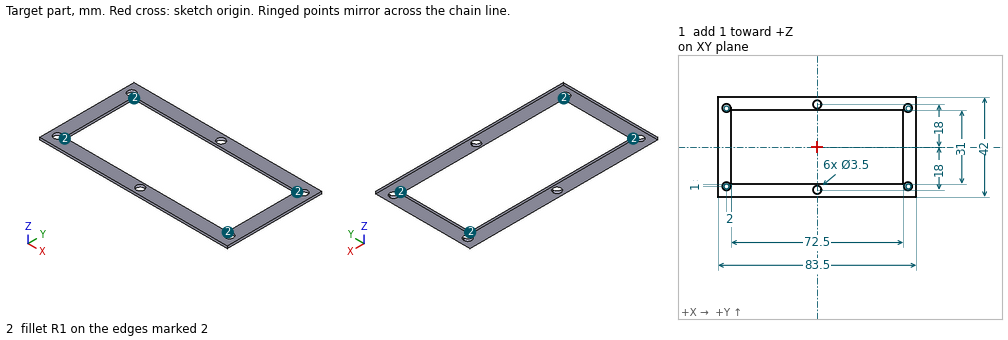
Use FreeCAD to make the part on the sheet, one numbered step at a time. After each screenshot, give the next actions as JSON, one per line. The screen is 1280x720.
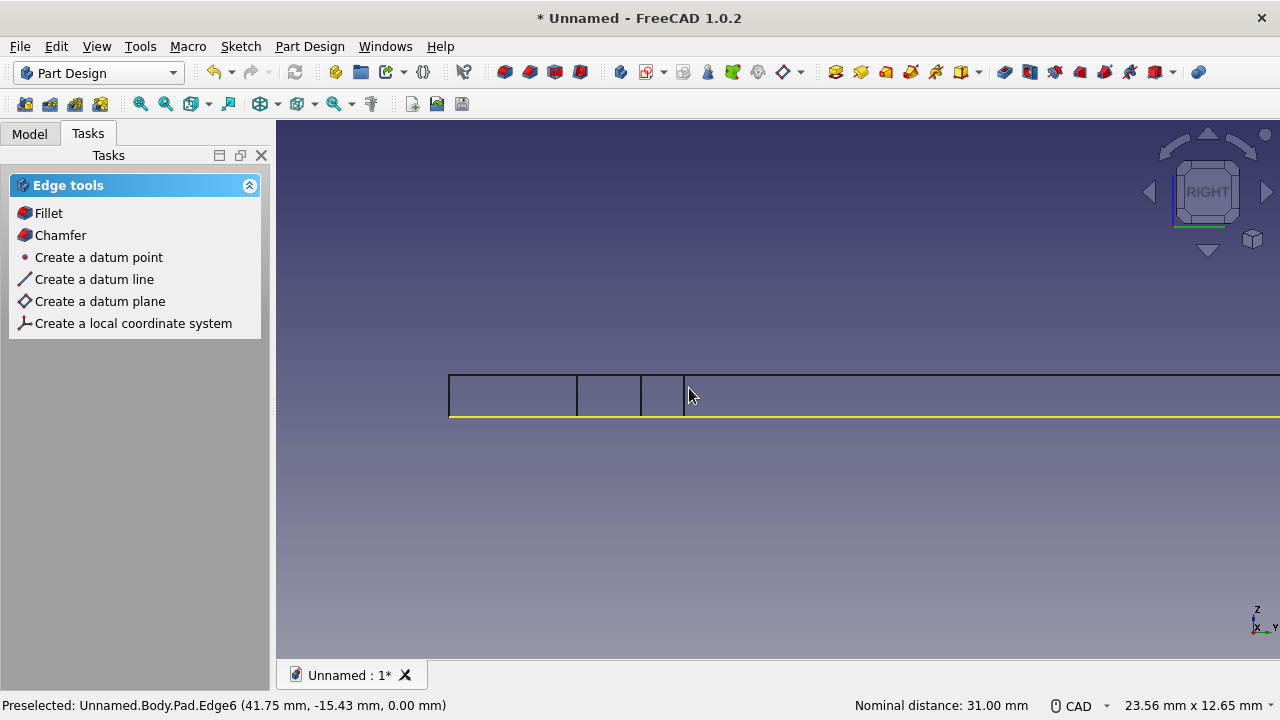
{"action": "left_click", "coordinate": [684, 395], "text": "ctrl"}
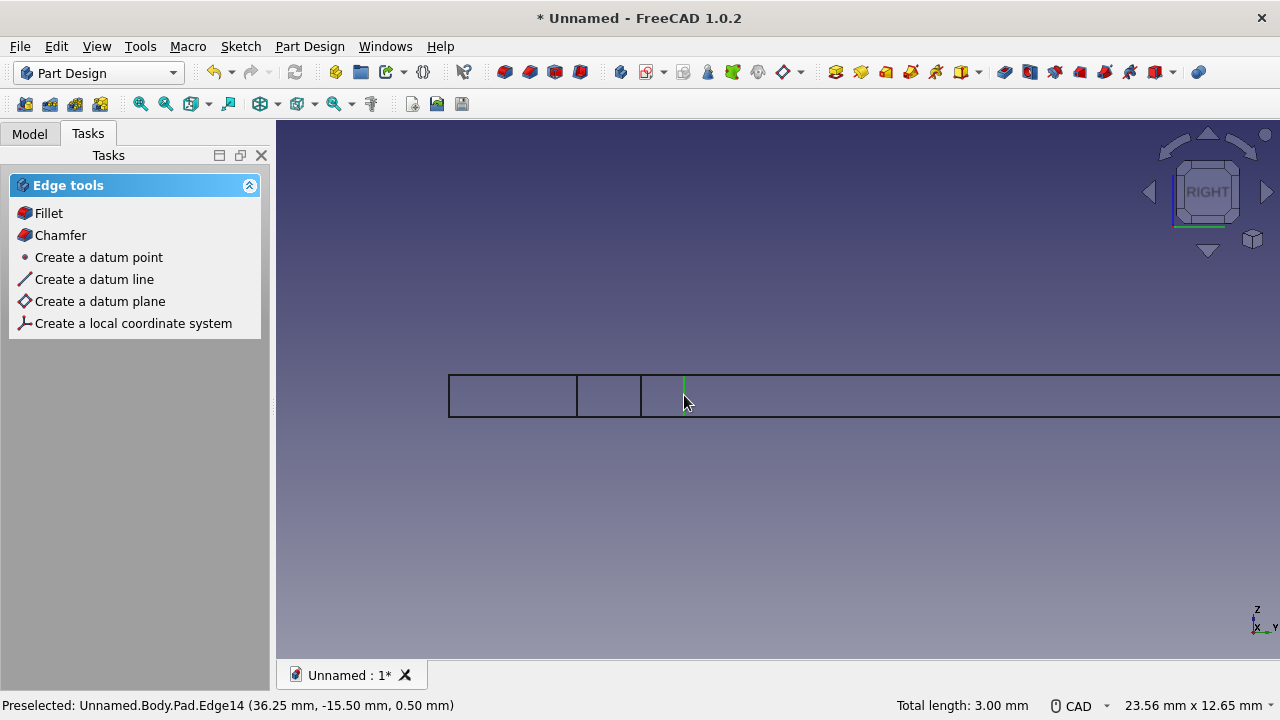
{"action": "left_click", "coordinate": [141, 104]}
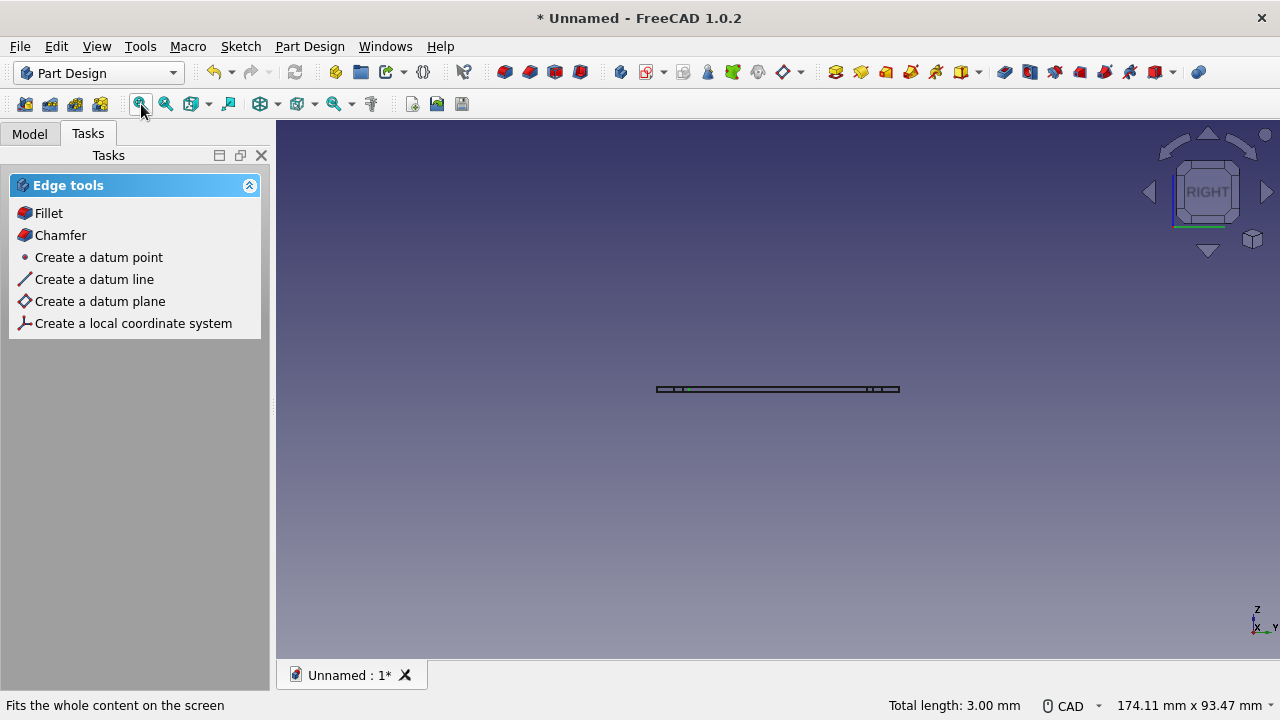
{"action": "key", "text": "5"}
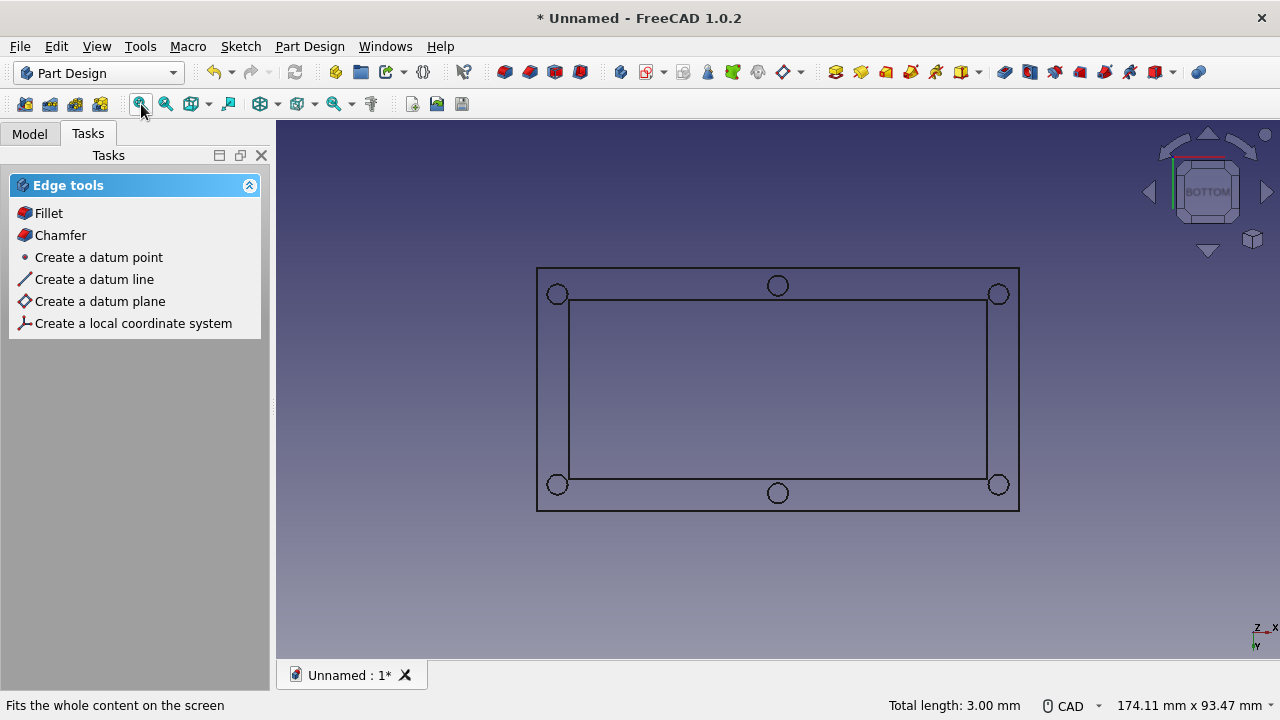
{"action": "scroll", "coordinate": [987, 478], "scroll_direction": "up", "scroll_amount": 10}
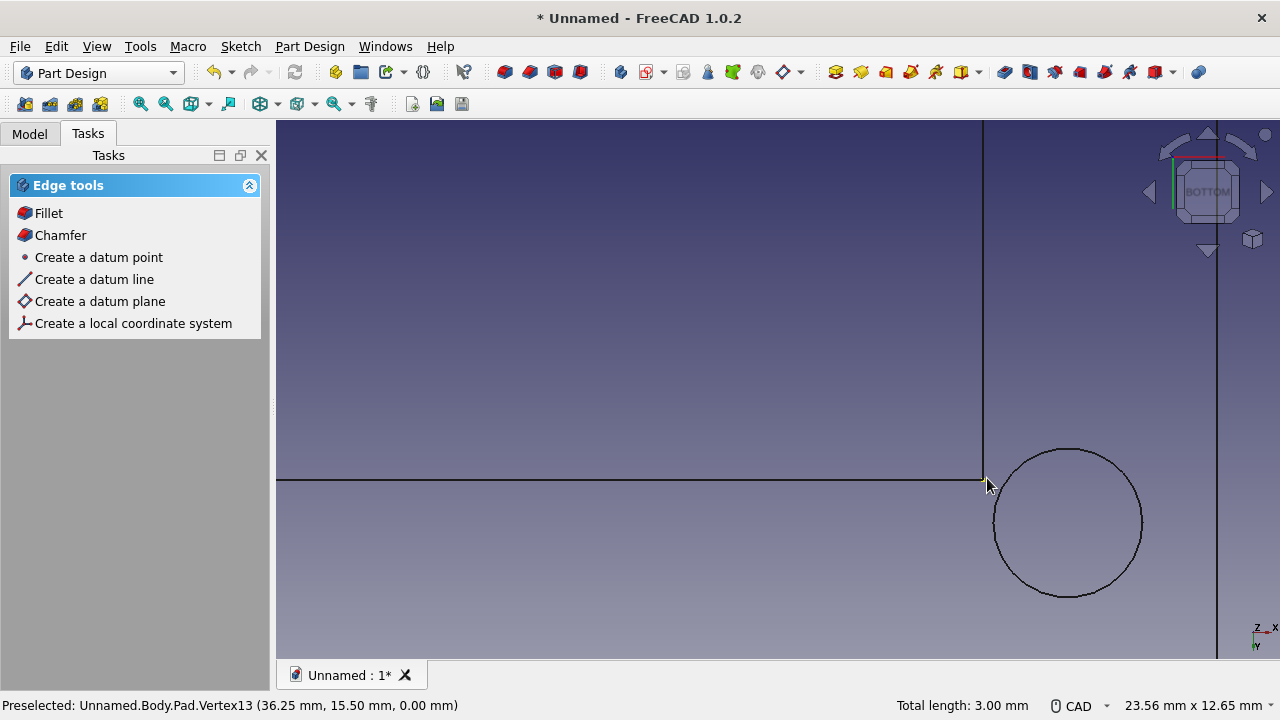
{"action": "key", "text": "v f"}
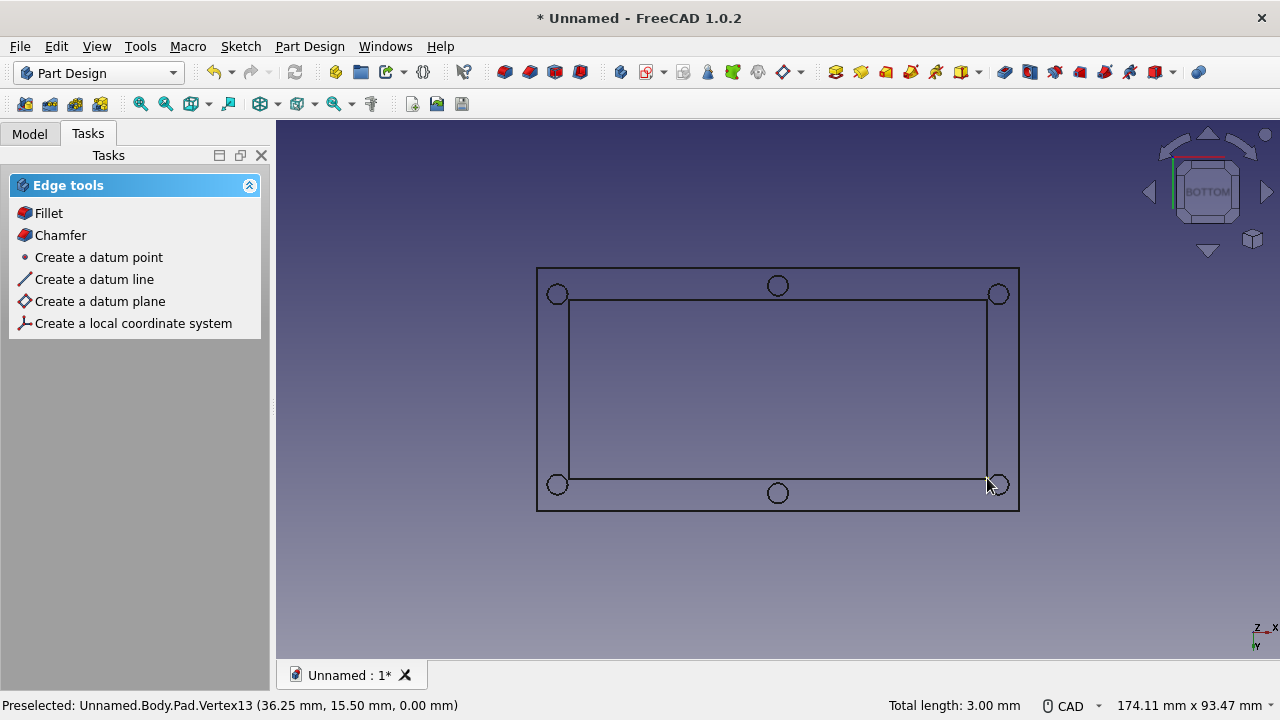
{"action": "key", "text": "4"}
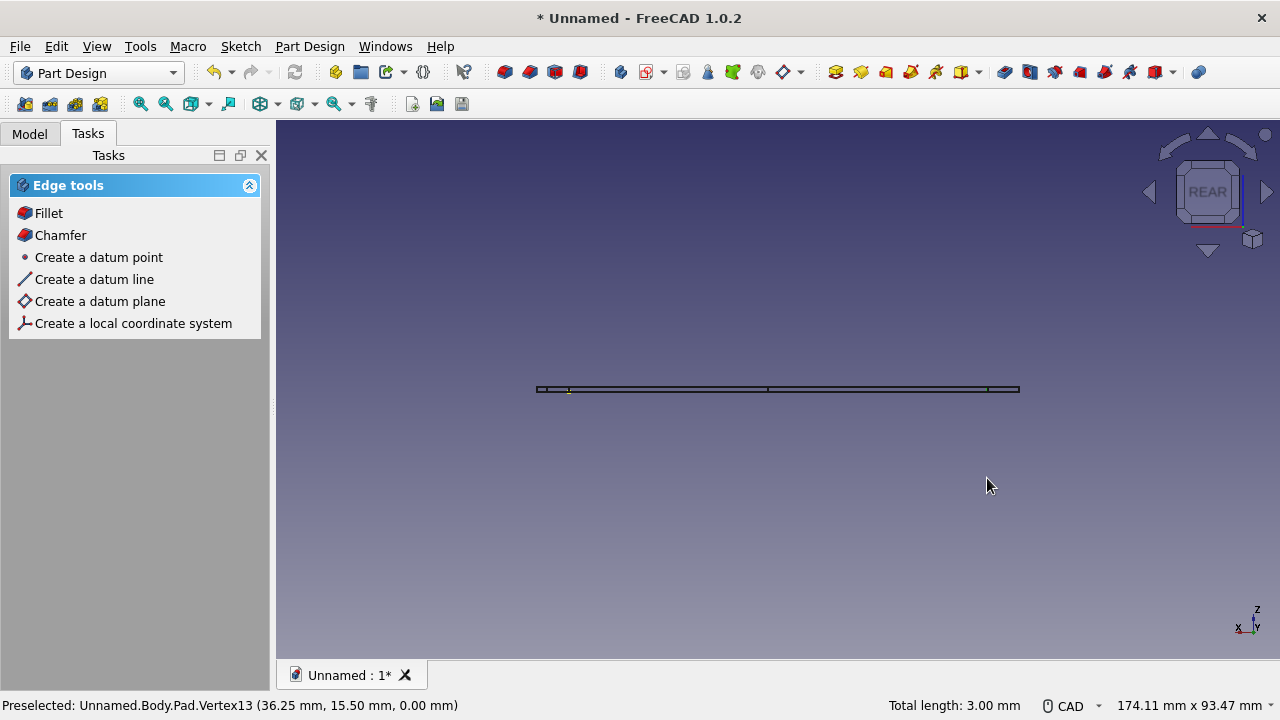
{"action": "scroll", "coordinate": [569, 389], "scroll_direction": "up", "scroll_amount": 10}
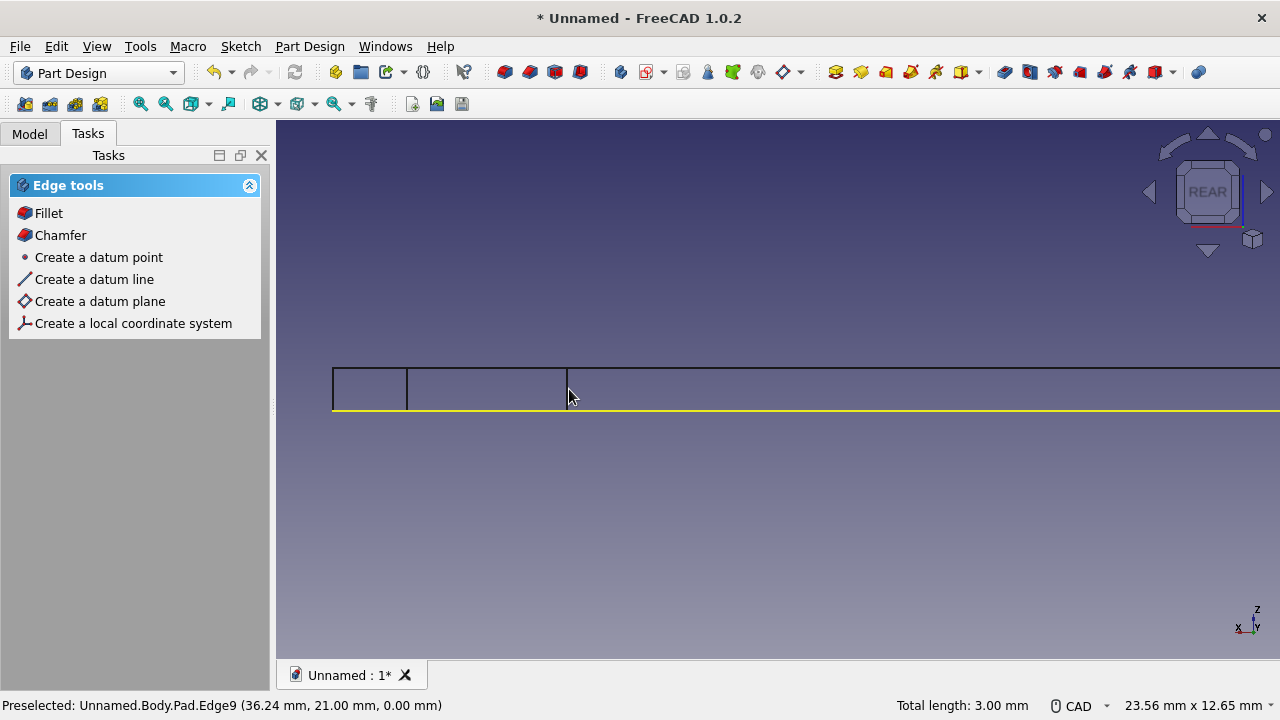
{"action": "left_click", "coordinate": [567, 389], "text": "ctrl"}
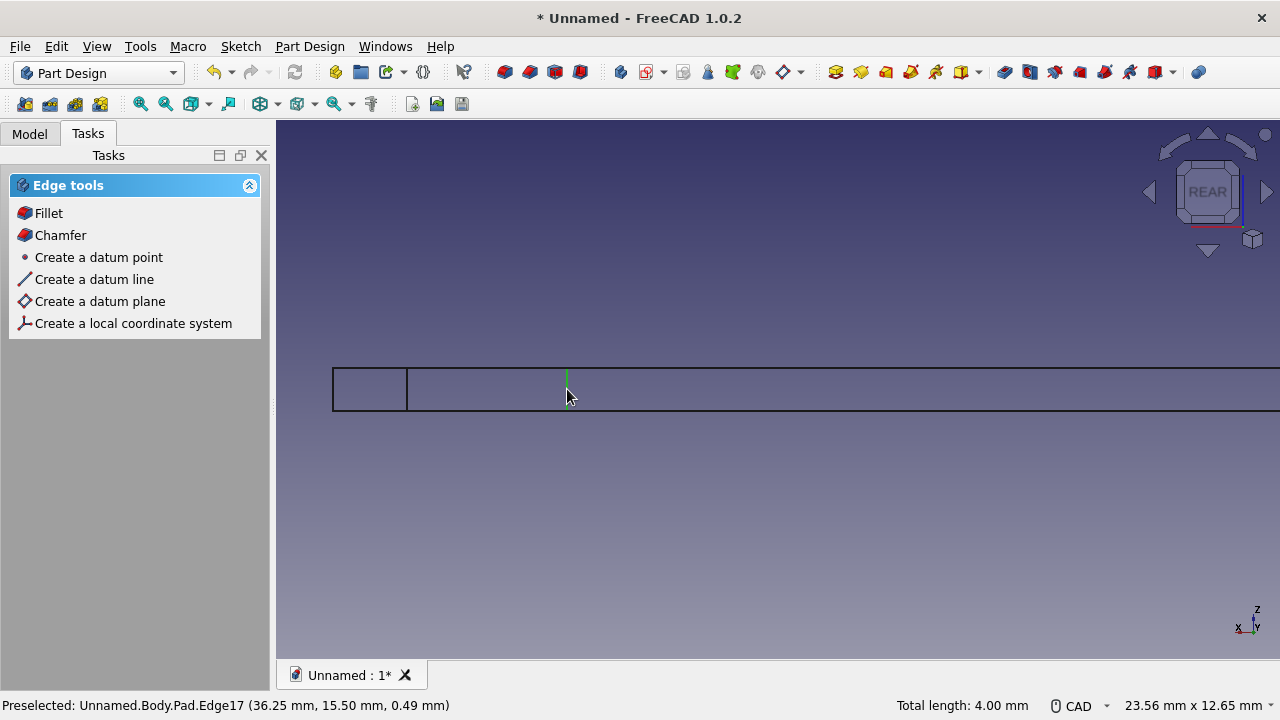
{"action": "key", "text": "v 1"}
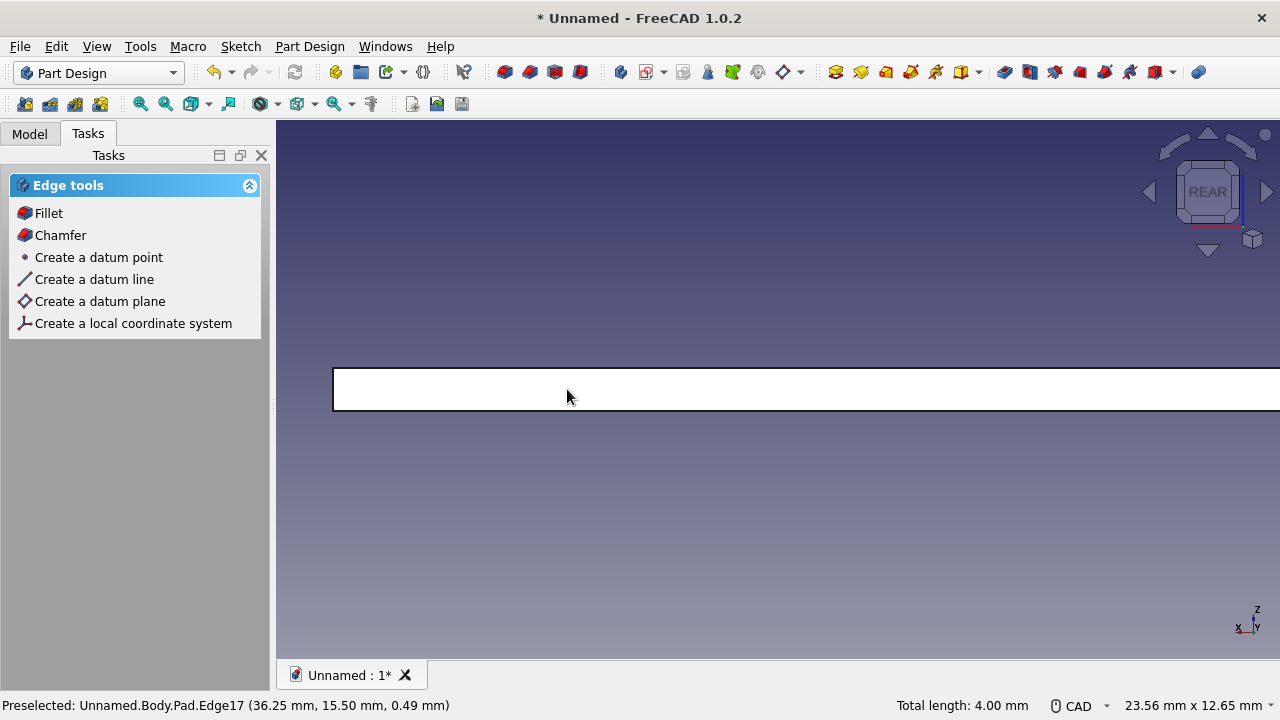
{"action": "left_click", "coordinate": [505, 72]}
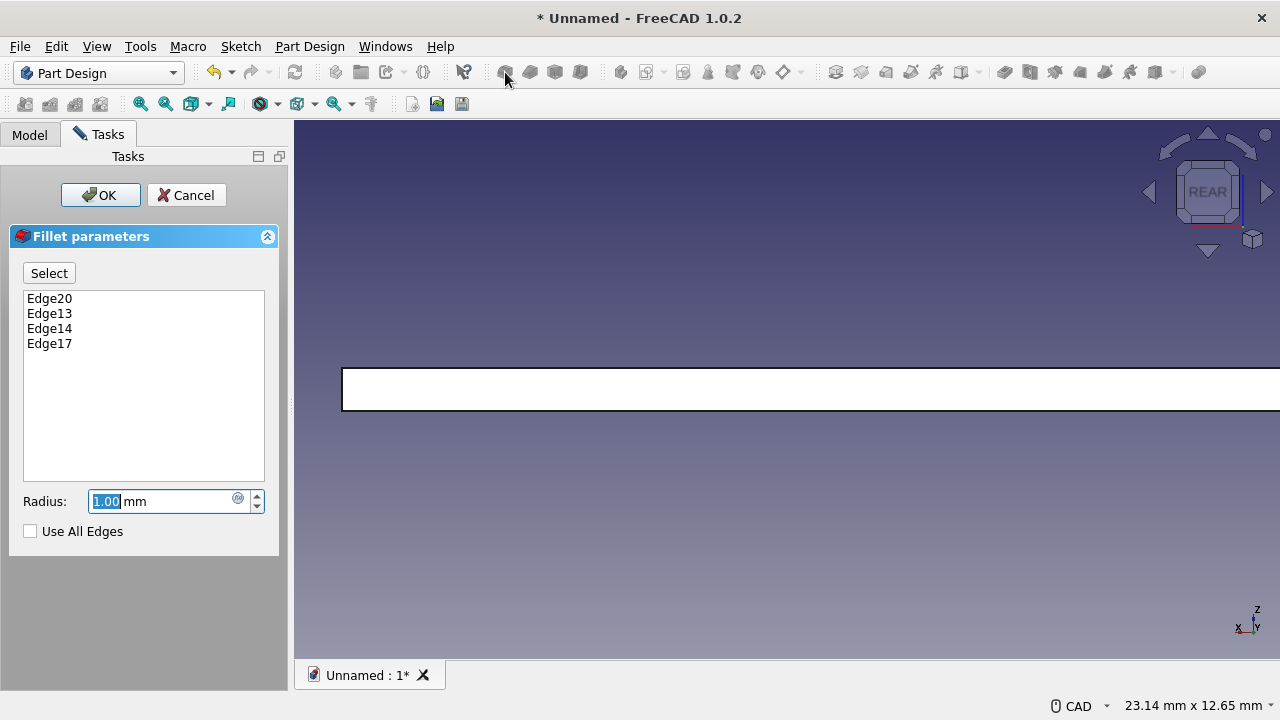
{"action": "type", "text": "1"}
{"action": "key", "text": "Tab"}